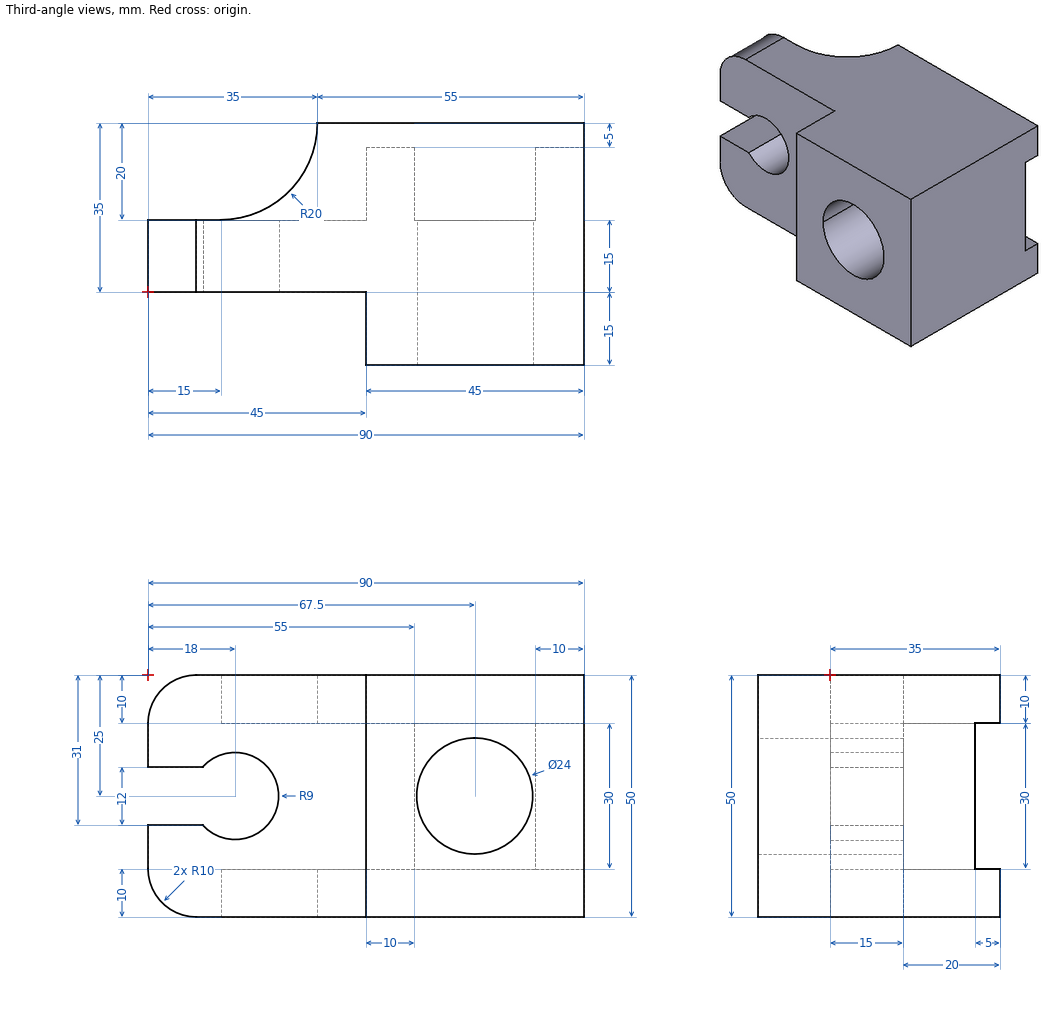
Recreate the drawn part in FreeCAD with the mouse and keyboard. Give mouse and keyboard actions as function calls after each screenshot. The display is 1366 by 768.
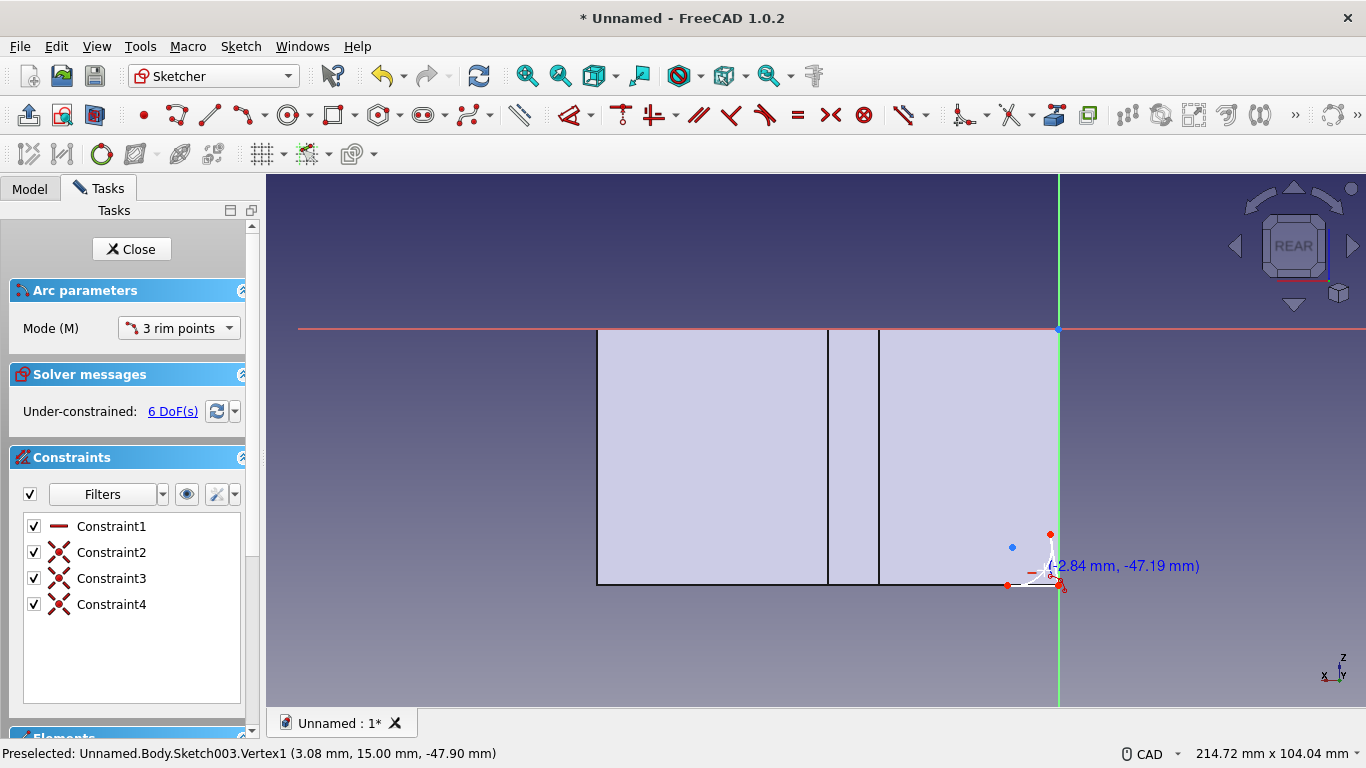
click(177, 116)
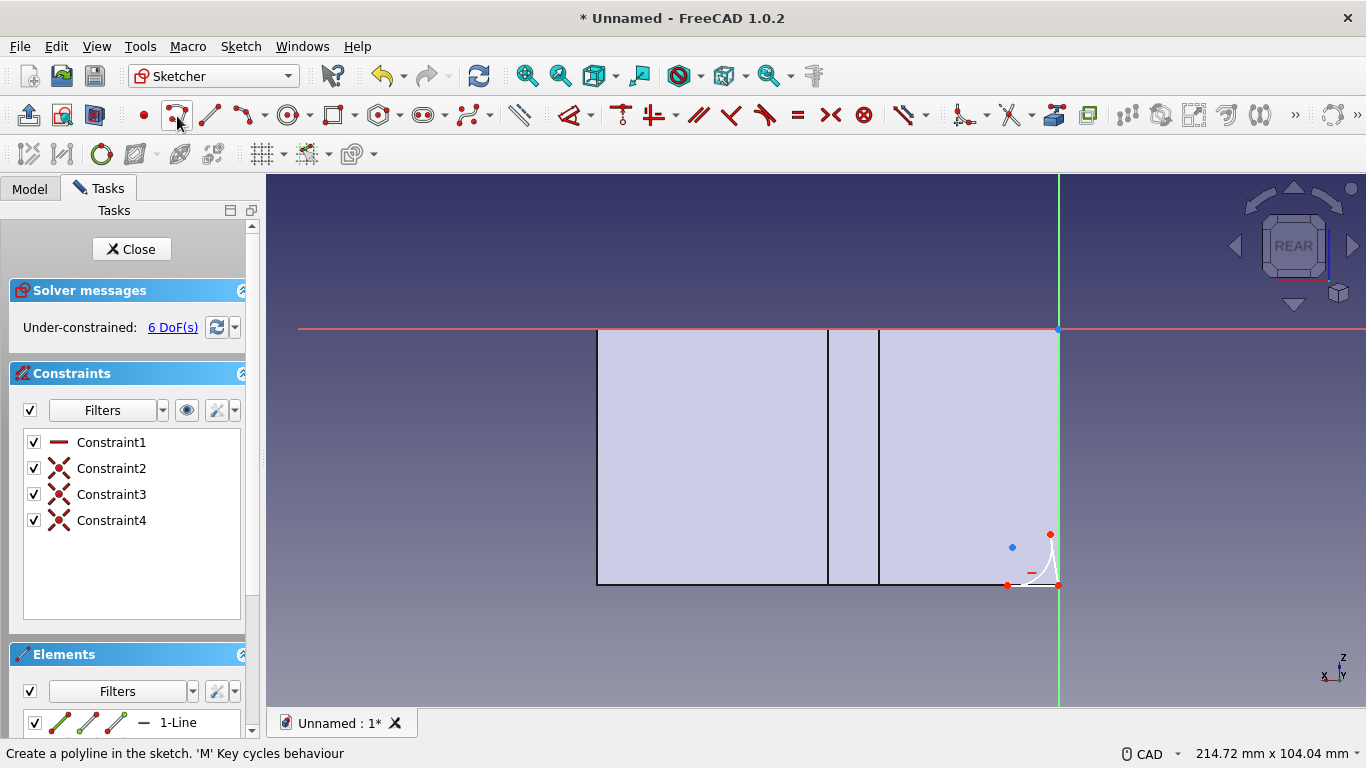
click(1059, 380)
click(1059, 329)
click(1007, 338)
right_click(1007, 338)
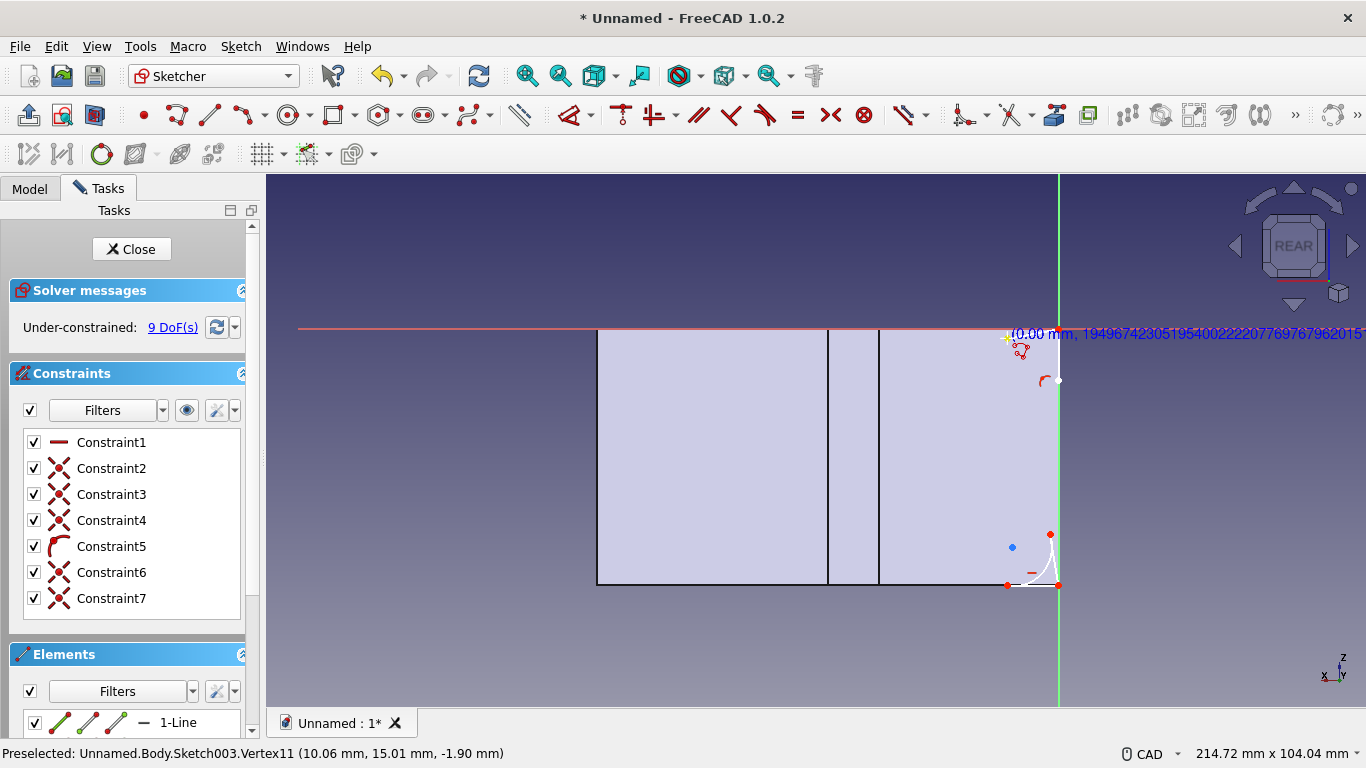
key(g)
key(3)
key(a)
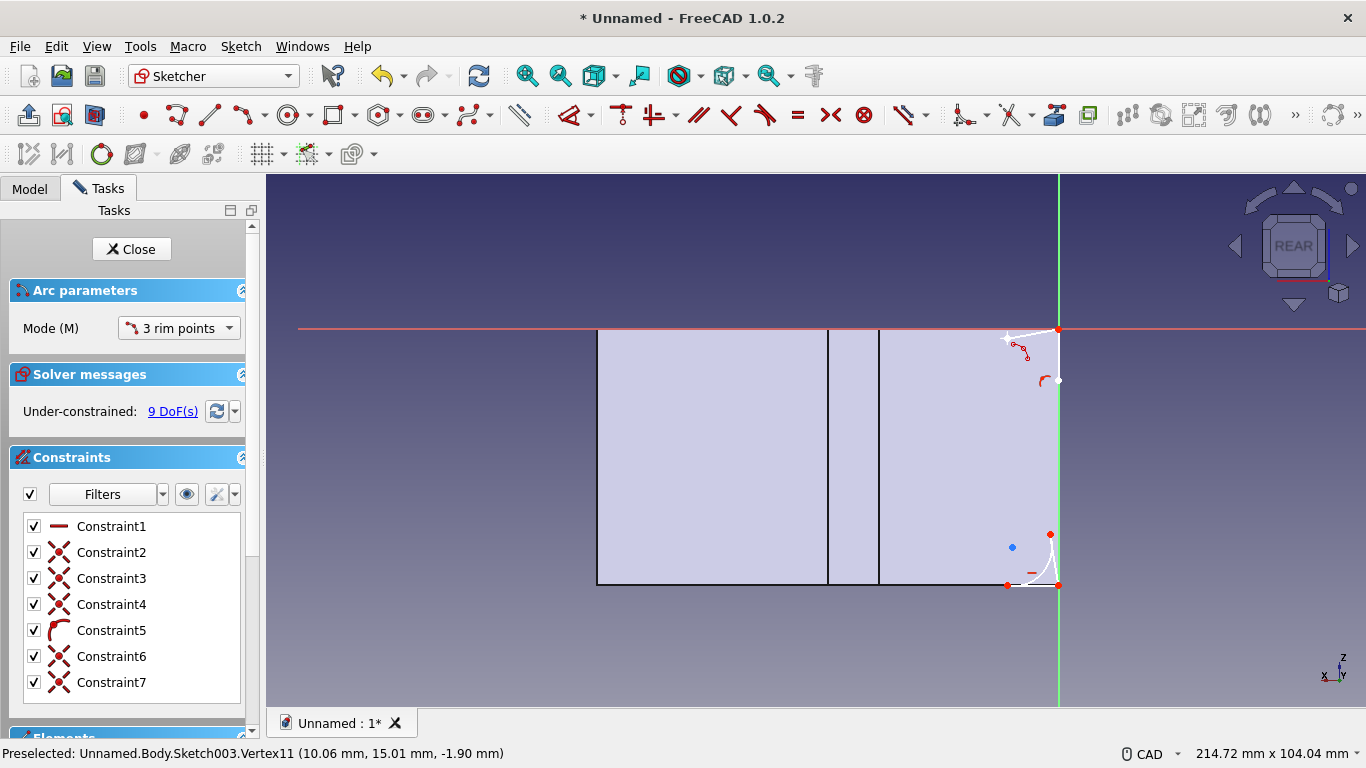
click(1007, 339)
click(1059, 381)
click(1044, 344)
key(Escape)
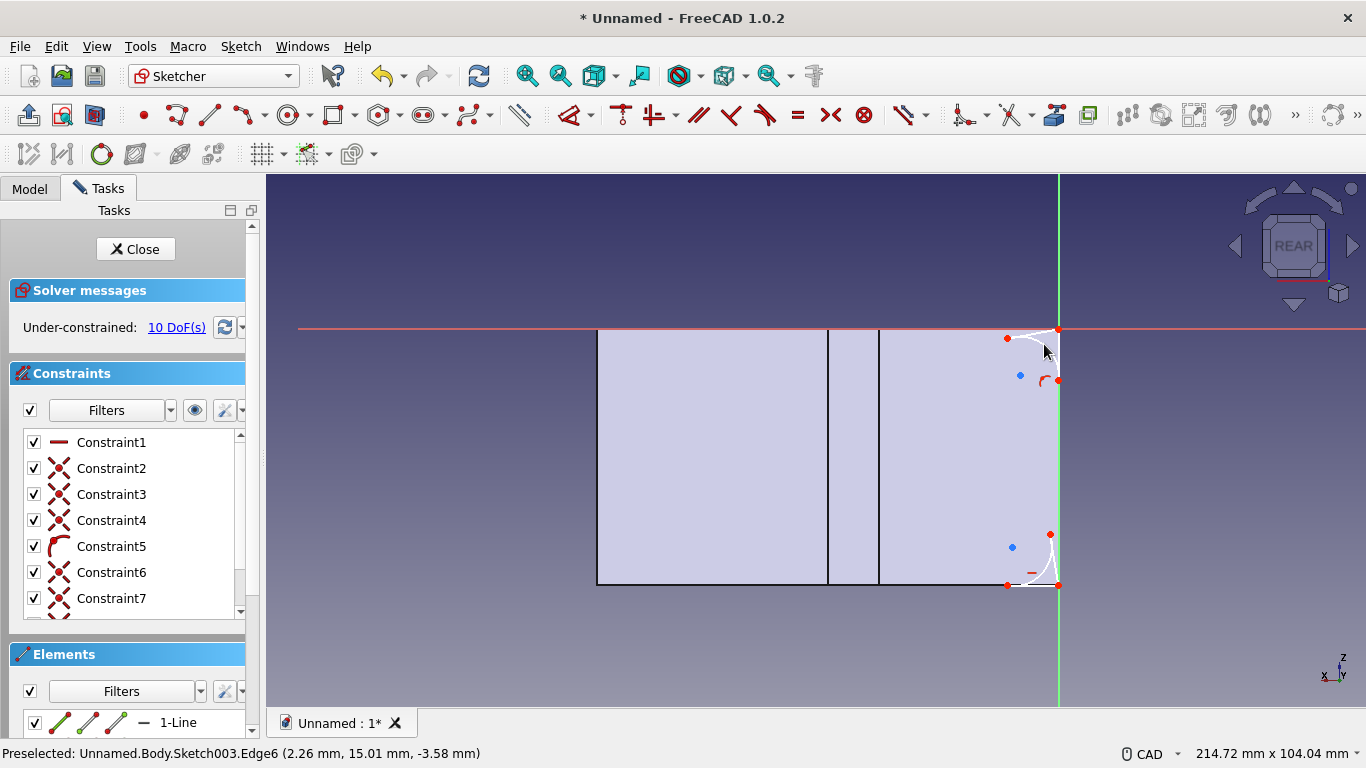
scroll(1043, 586, up, 2)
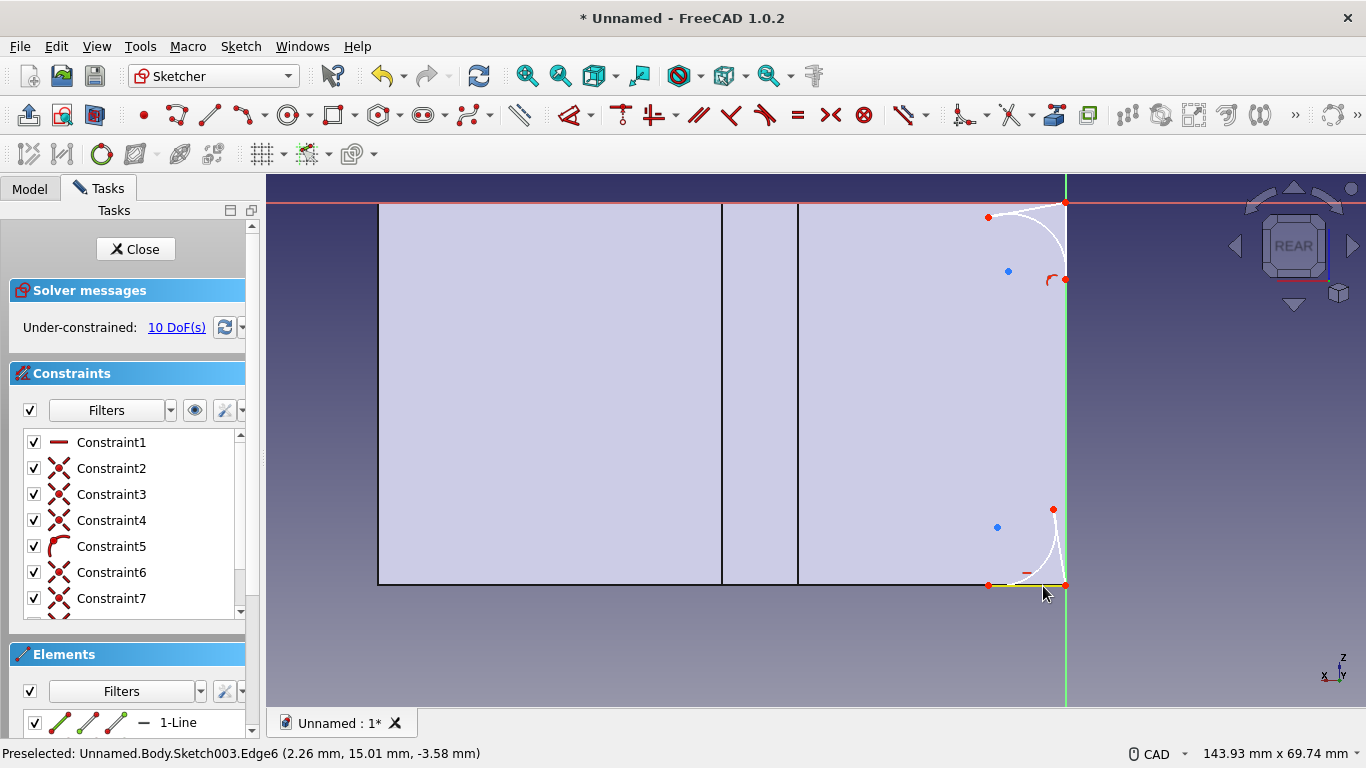
click(1043, 586)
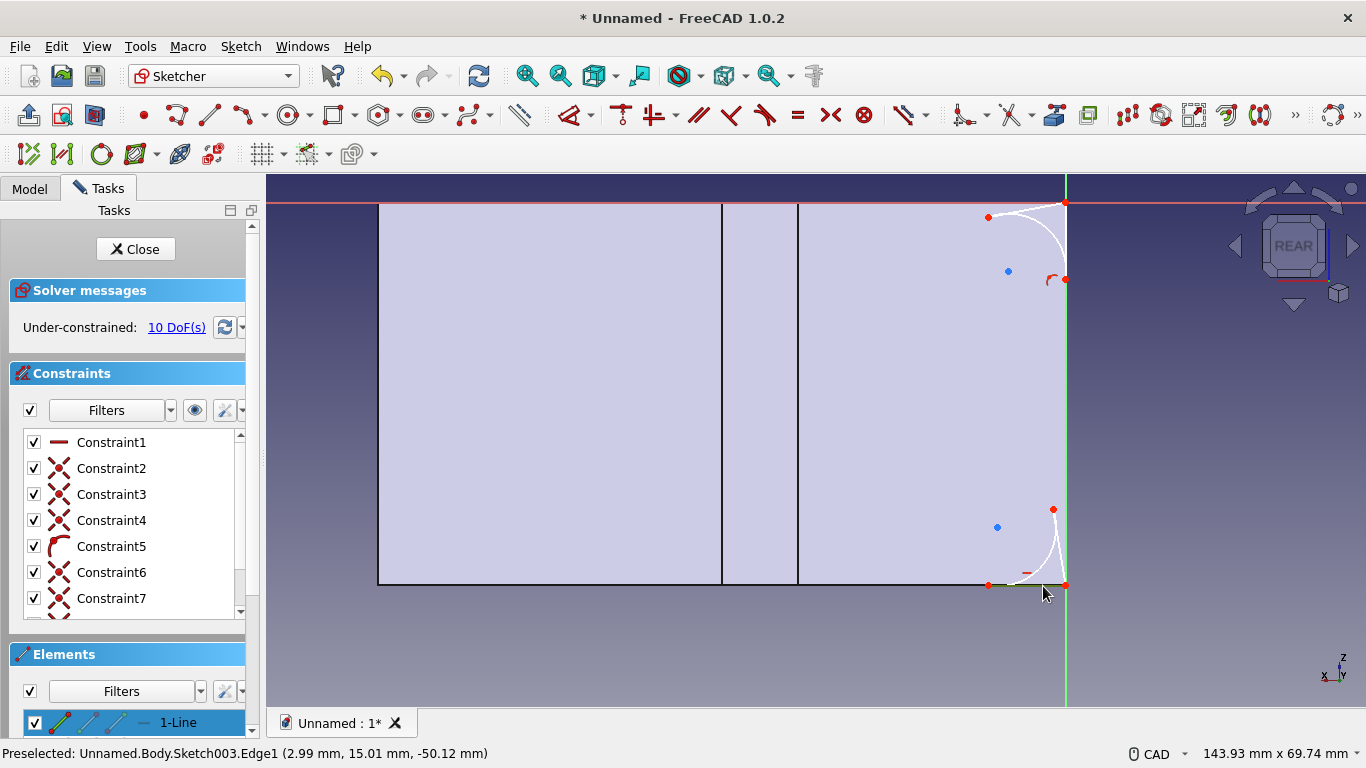
click(1042, 566)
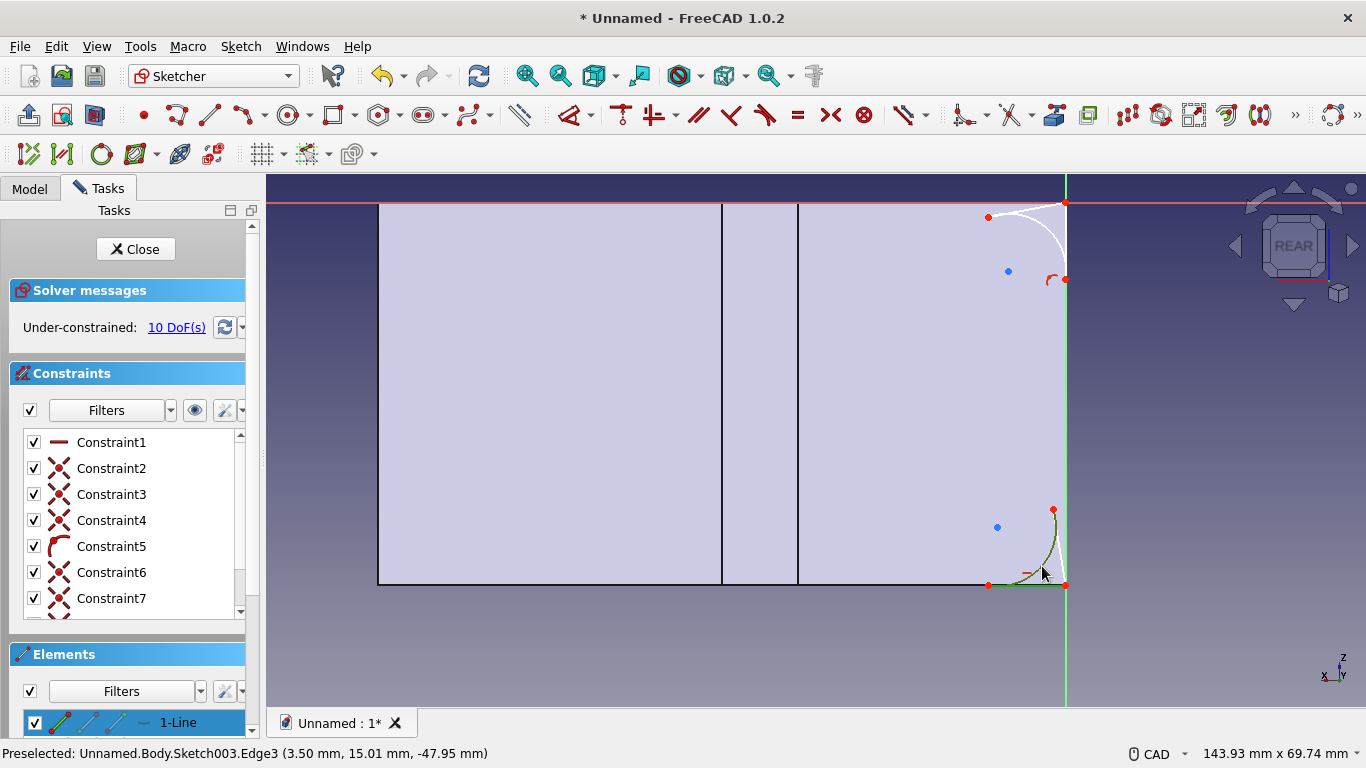
click(765, 116)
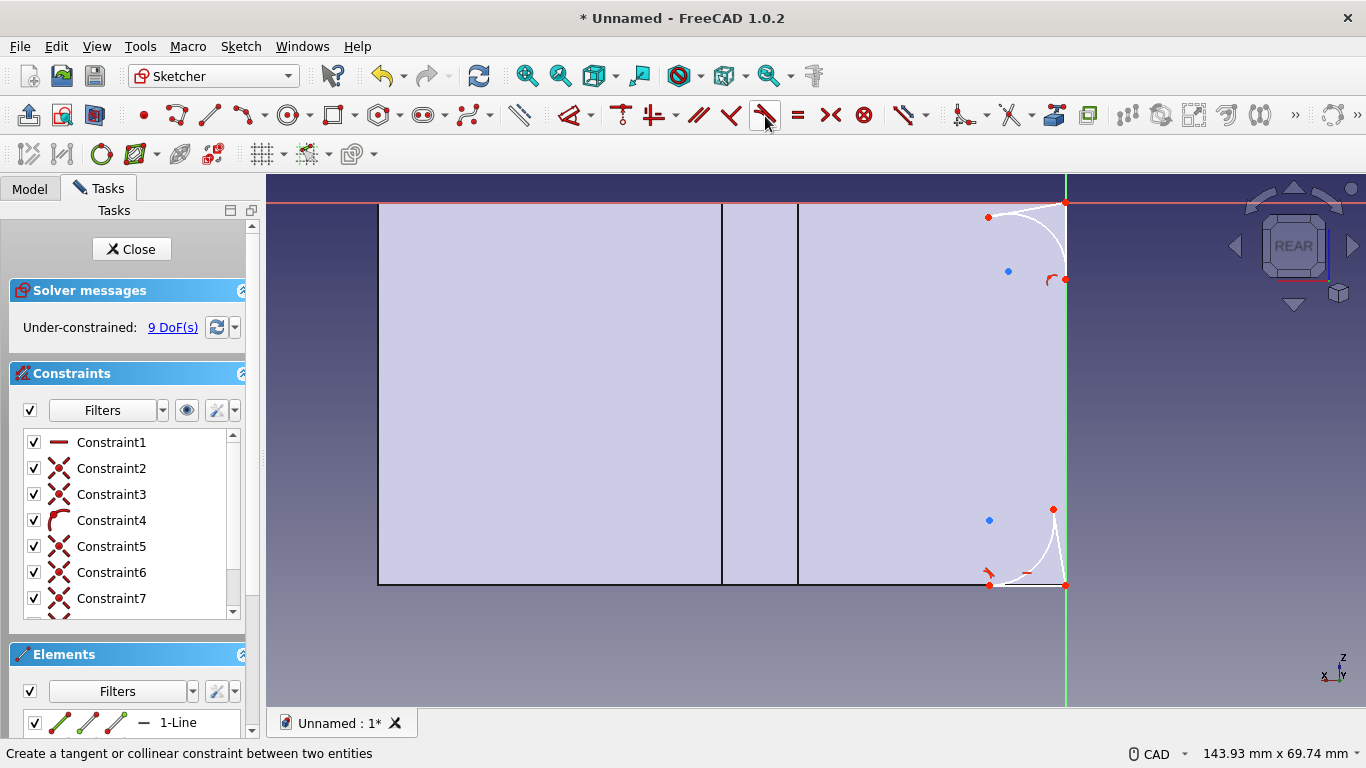
click(1062, 563)